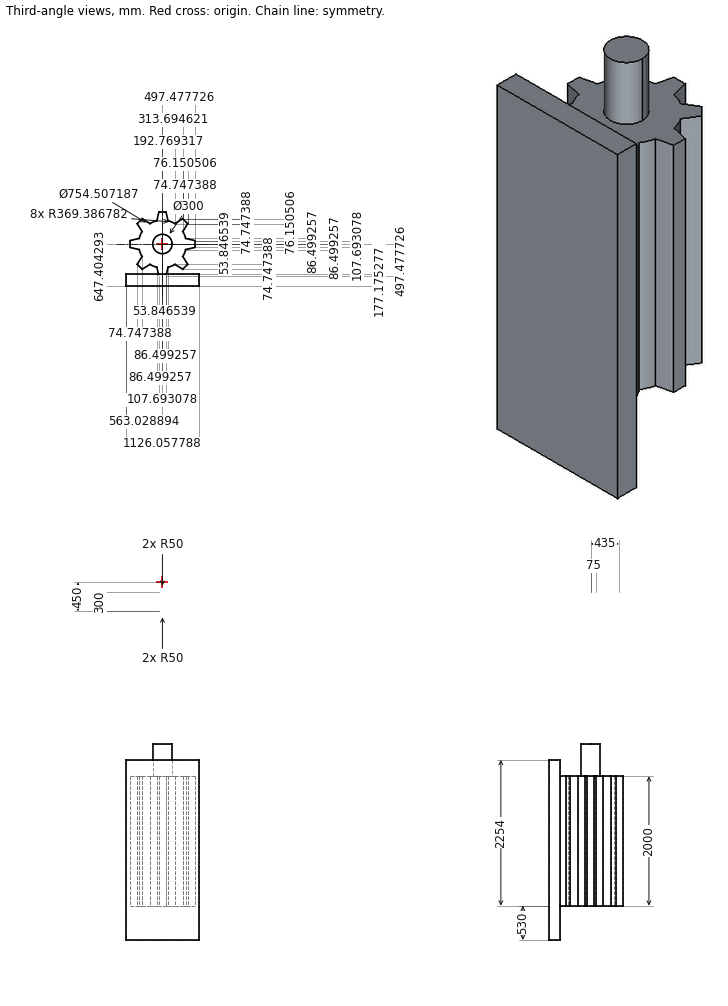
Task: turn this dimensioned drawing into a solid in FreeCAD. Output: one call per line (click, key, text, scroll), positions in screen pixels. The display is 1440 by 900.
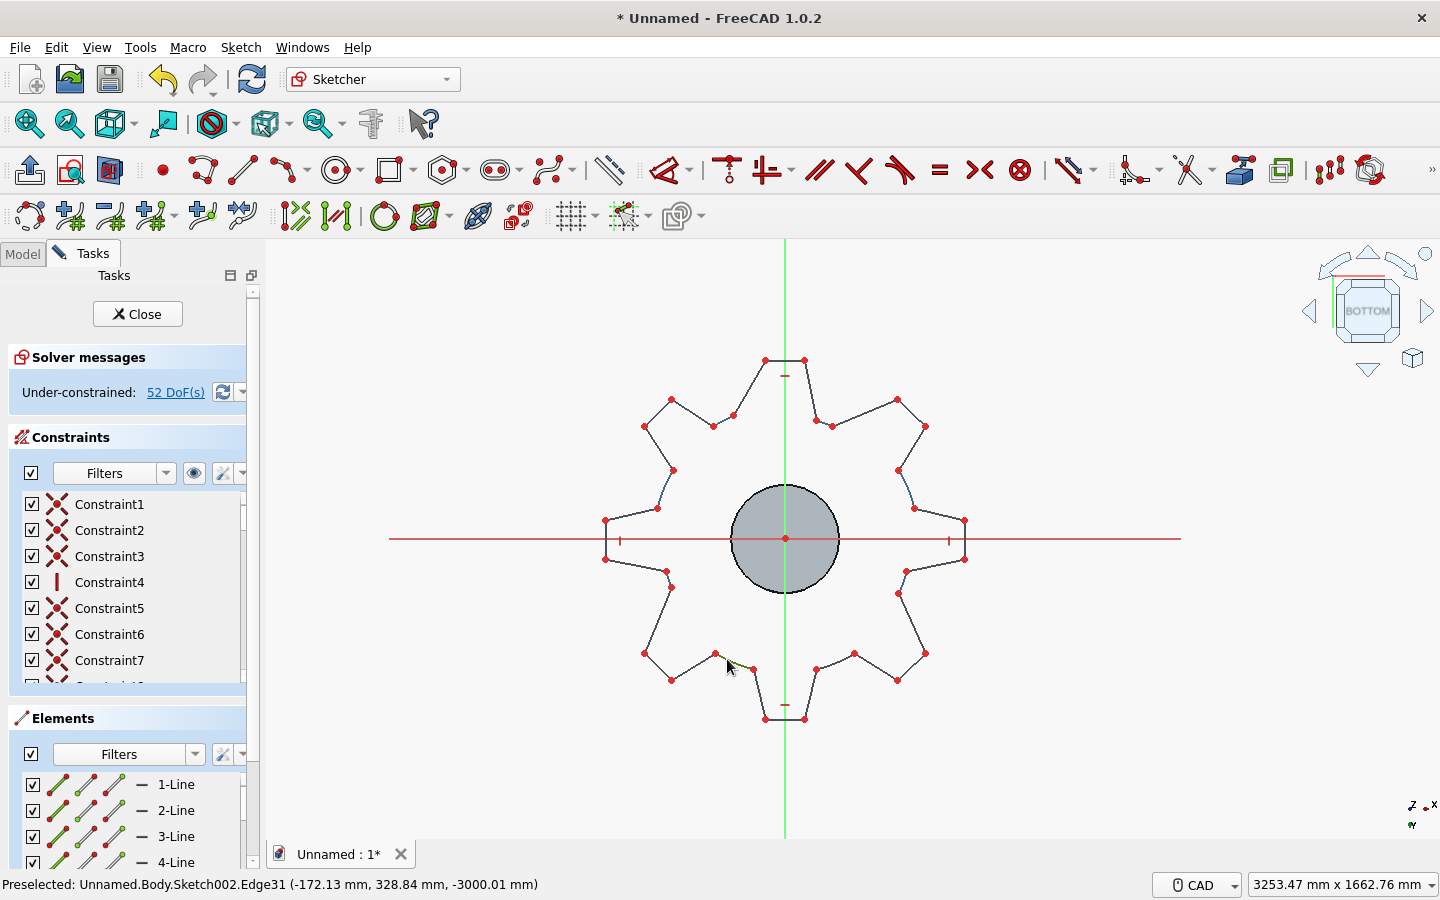
click(829, 666)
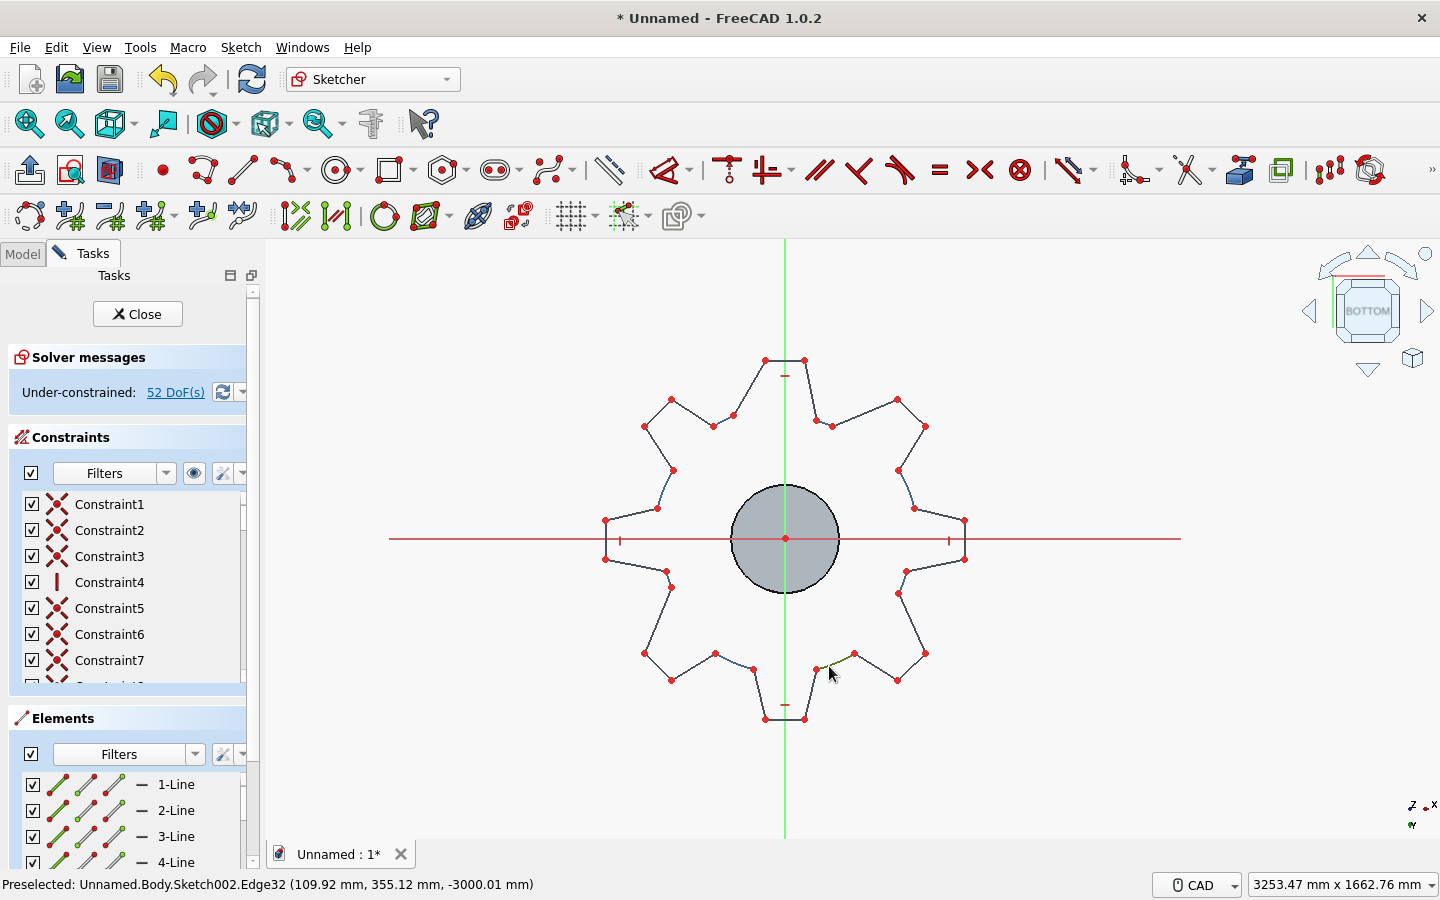
click(940, 170)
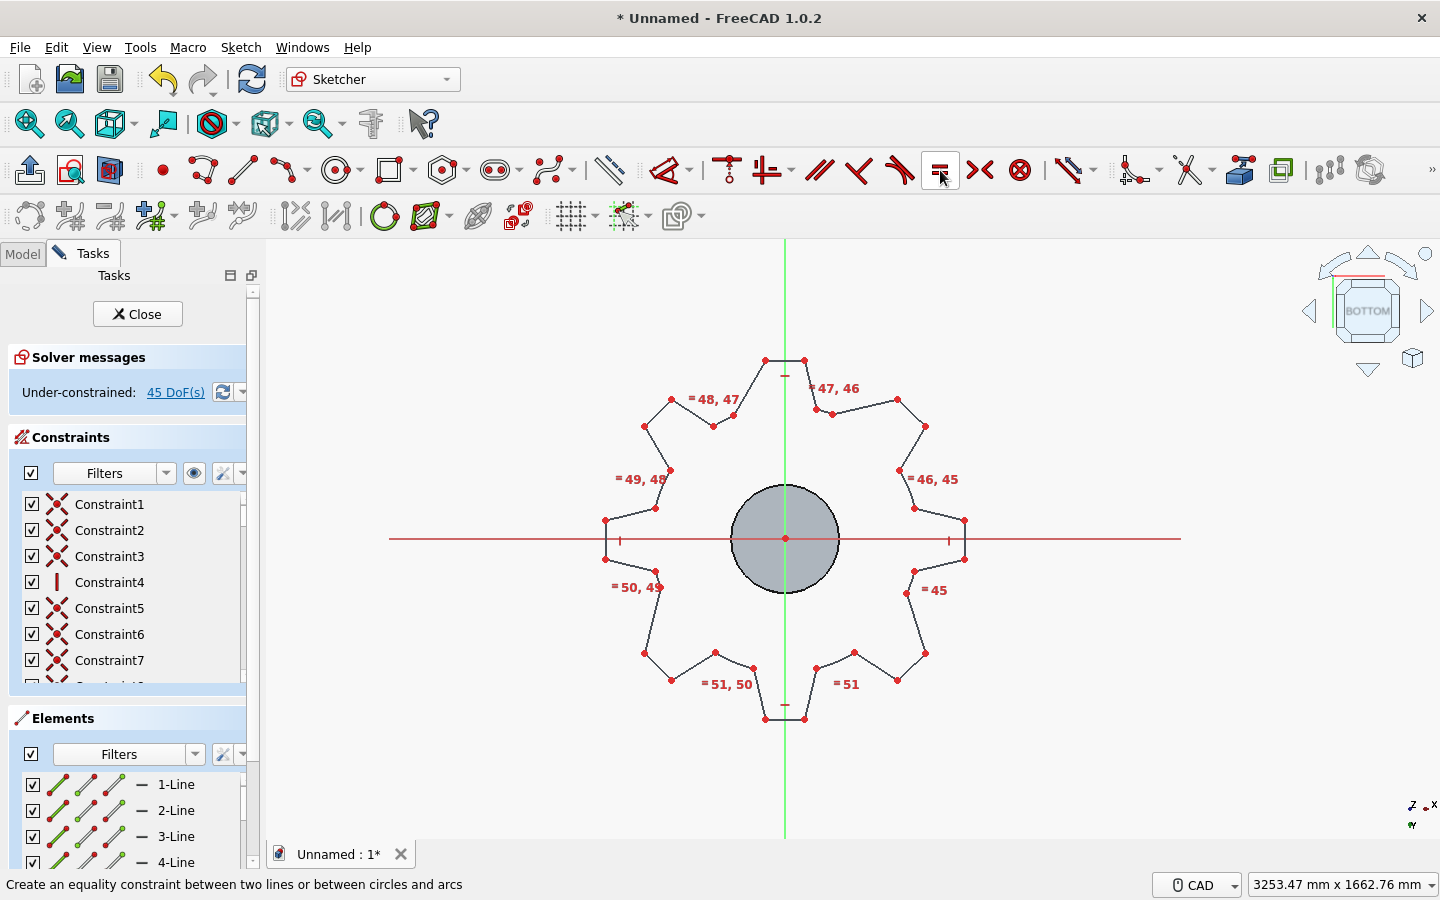
click(926, 654)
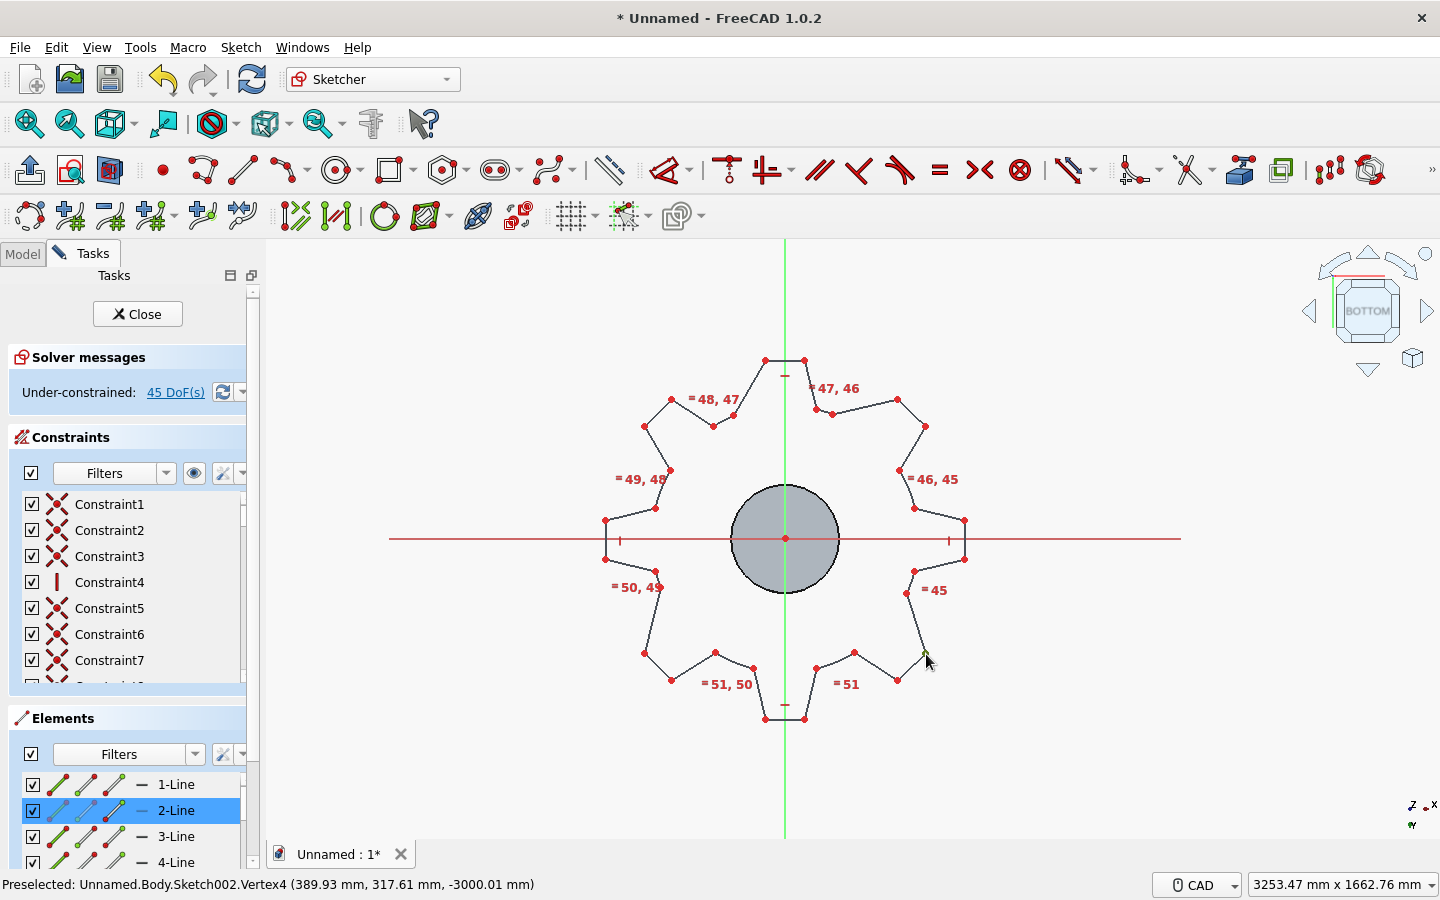
click(926, 427)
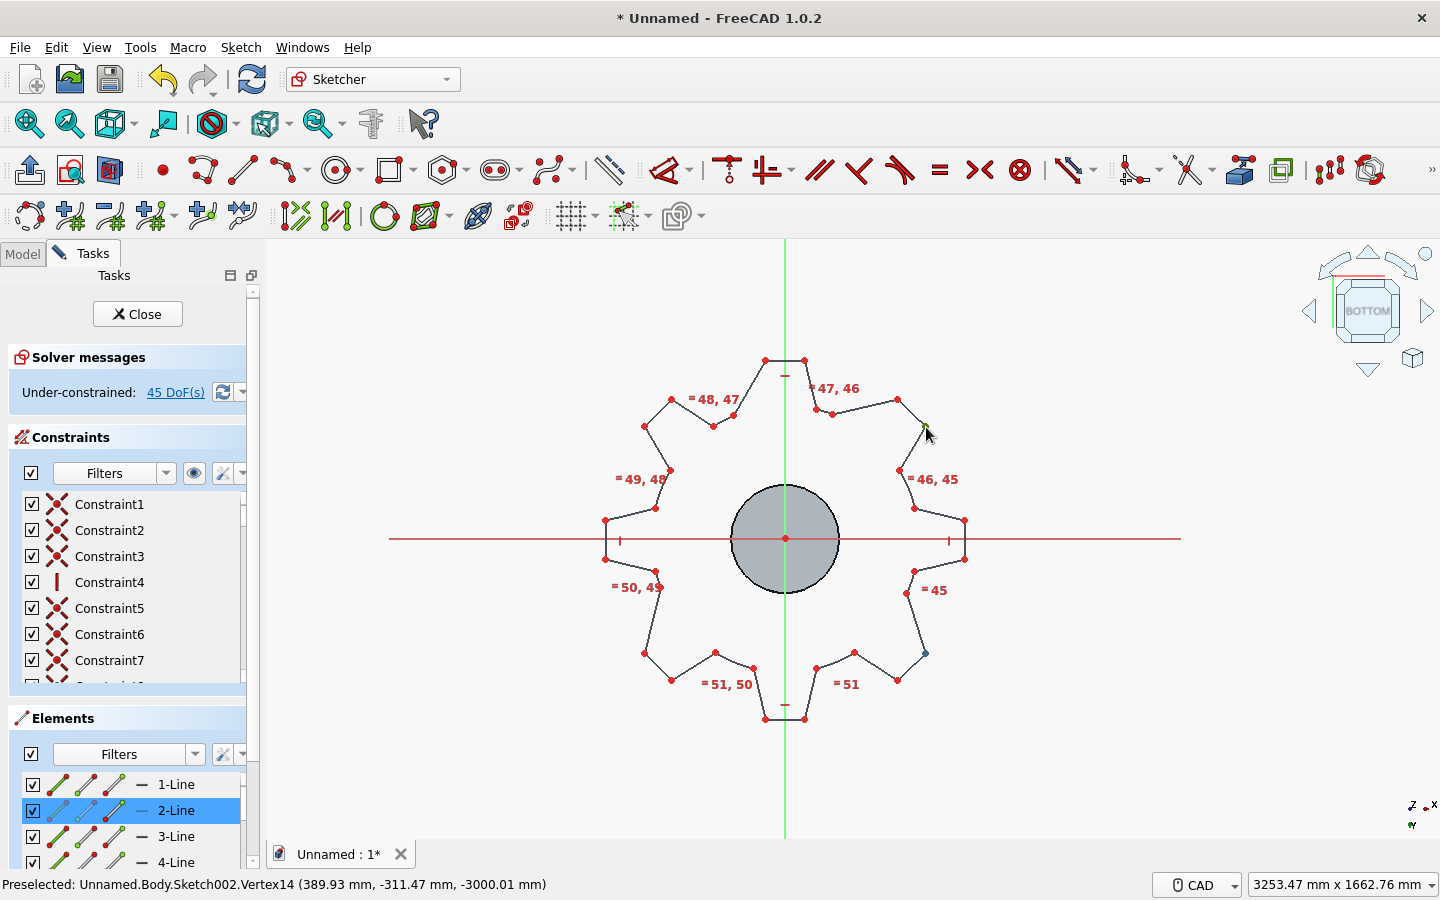
click(434, 539)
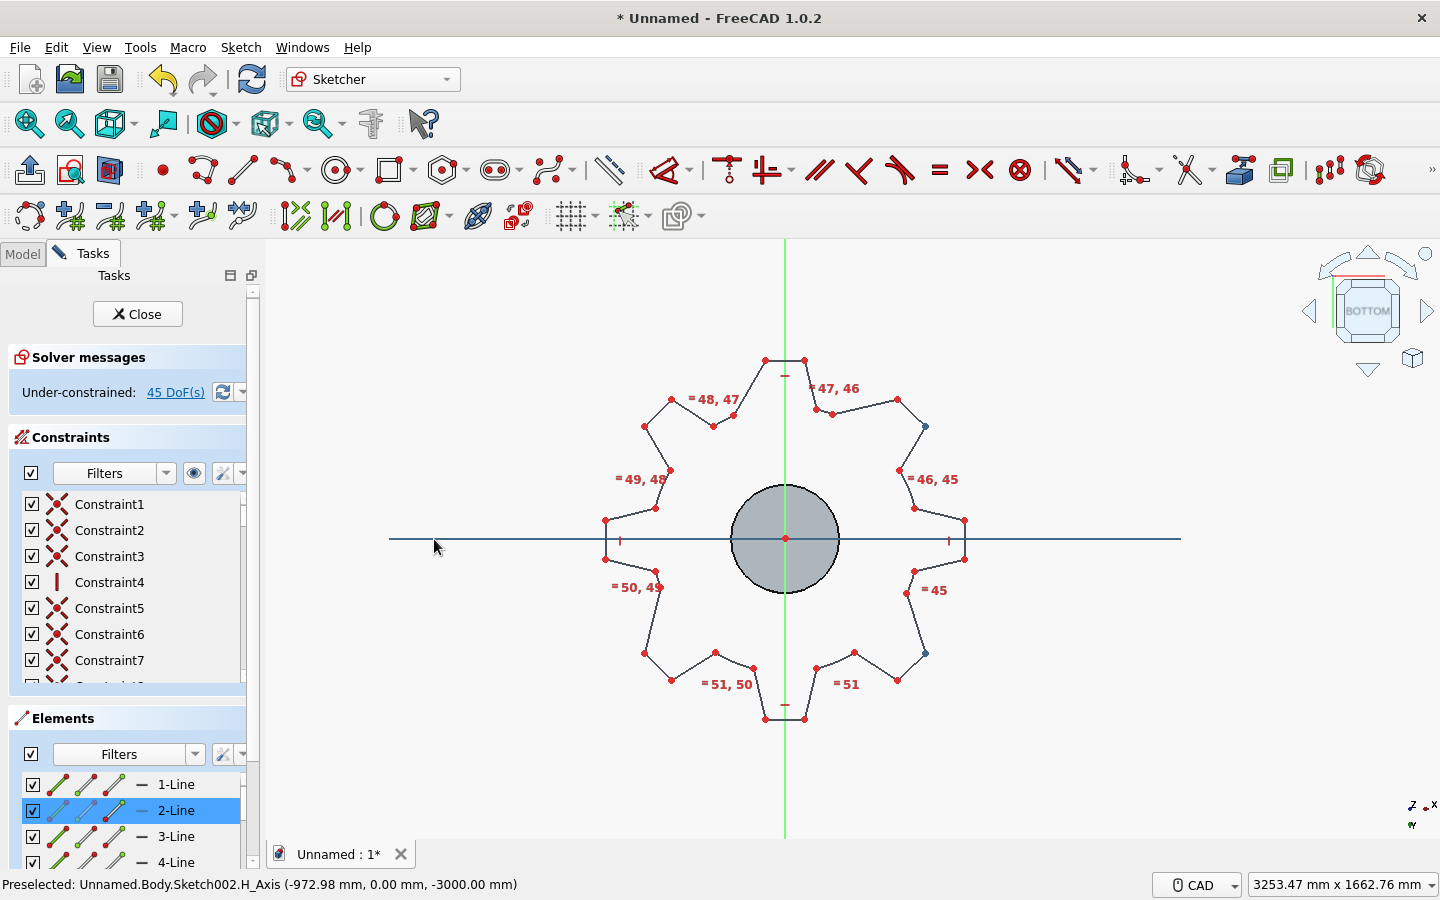
click(980, 170)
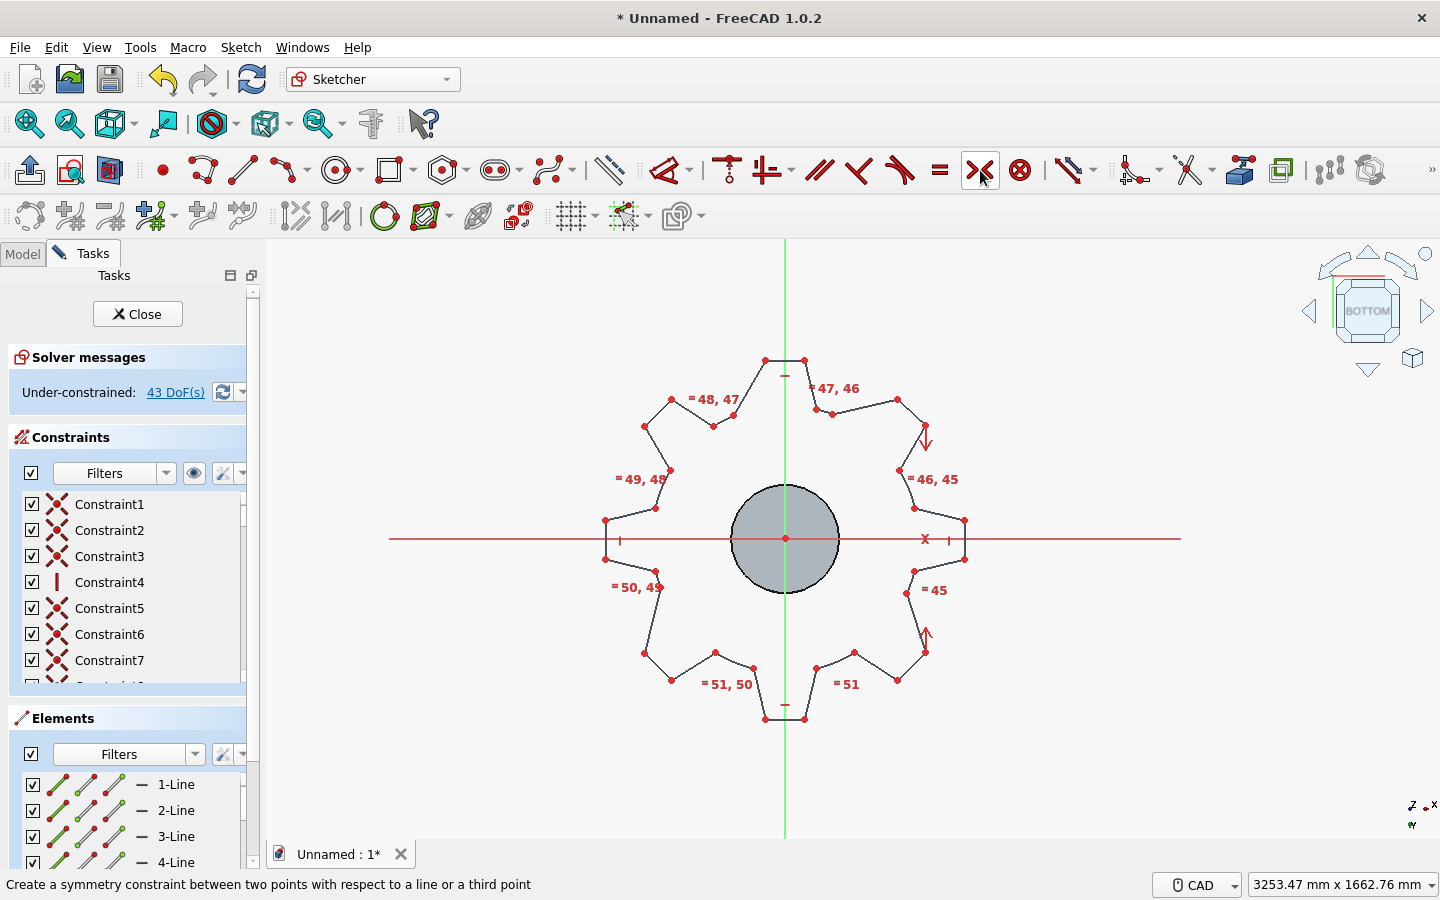
click(898, 681)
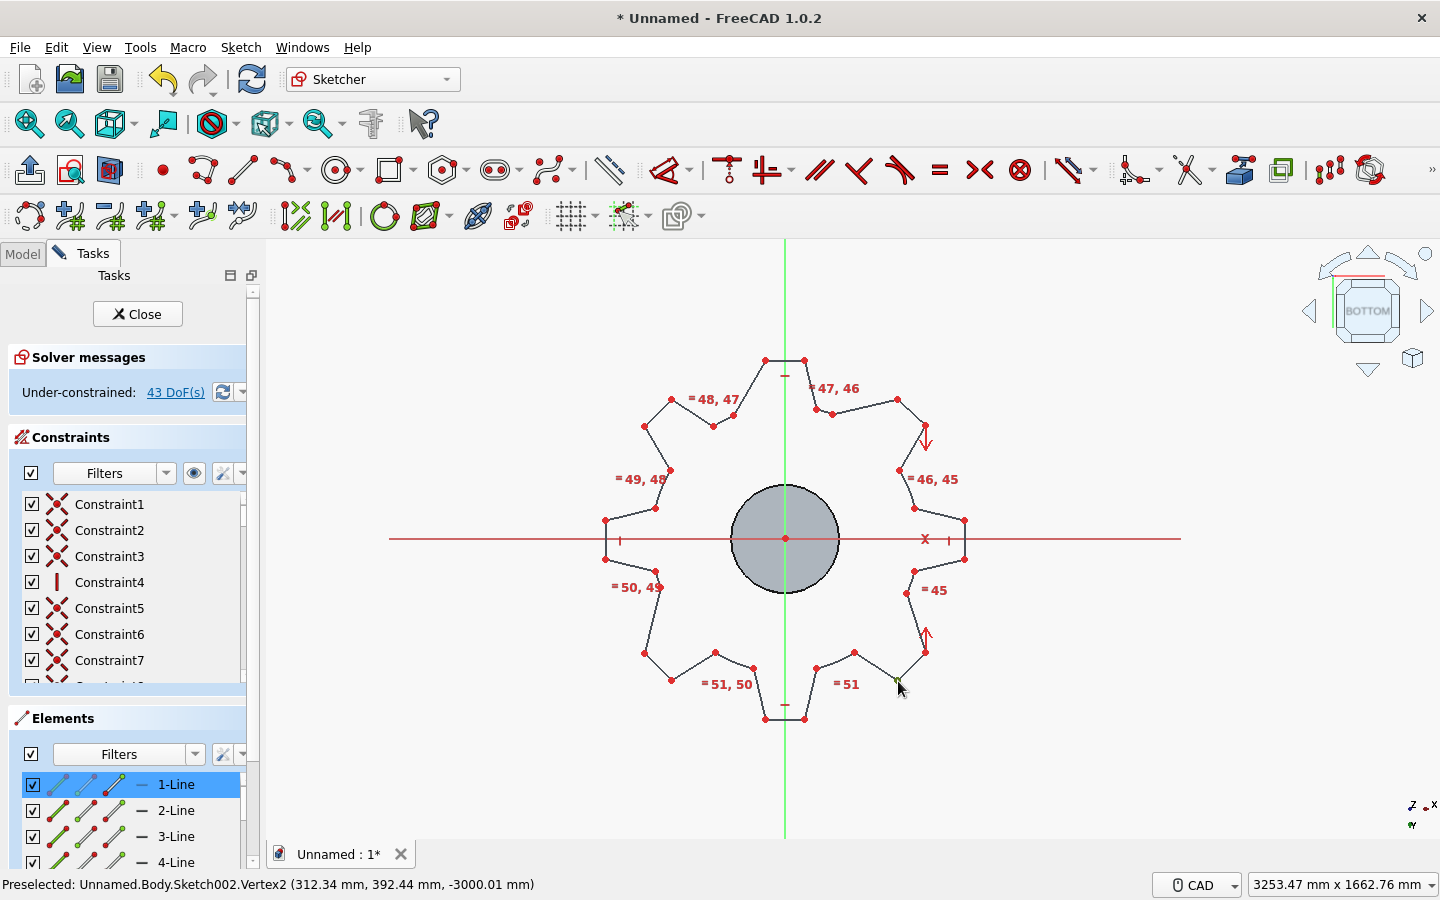
click(898, 400)